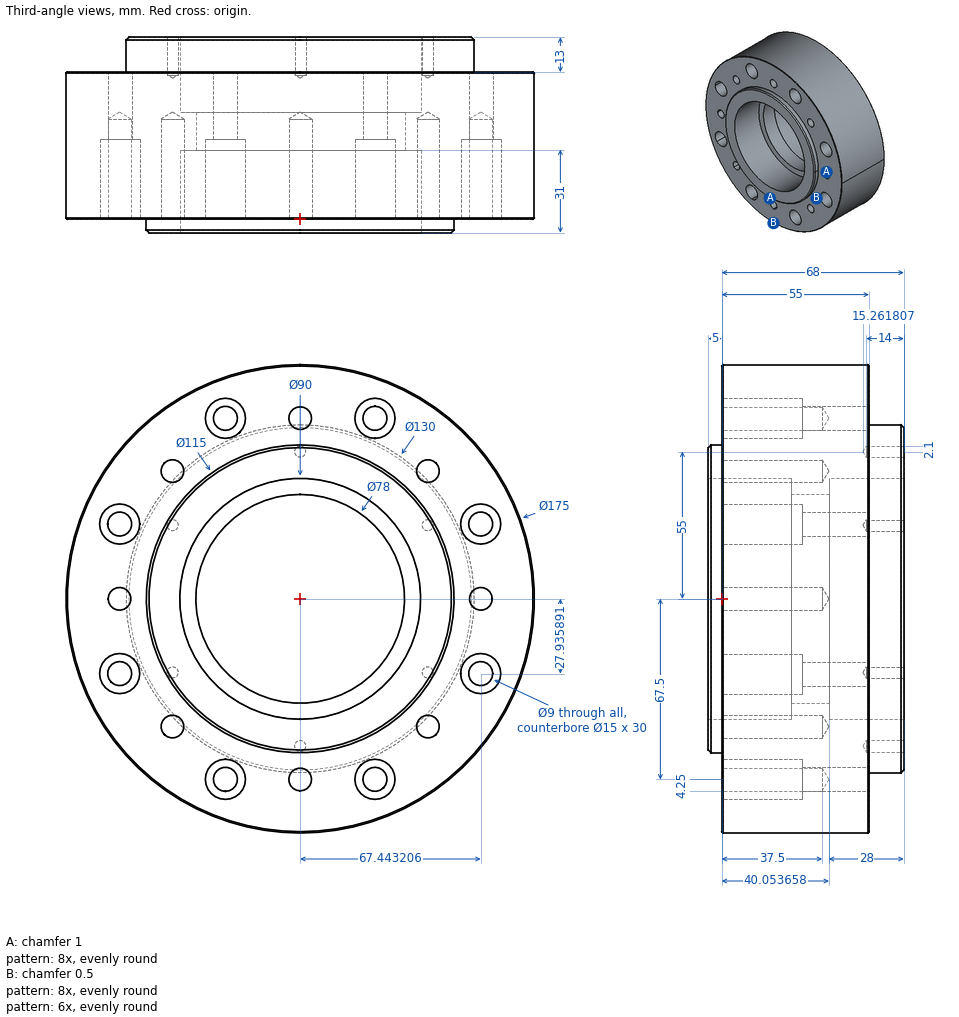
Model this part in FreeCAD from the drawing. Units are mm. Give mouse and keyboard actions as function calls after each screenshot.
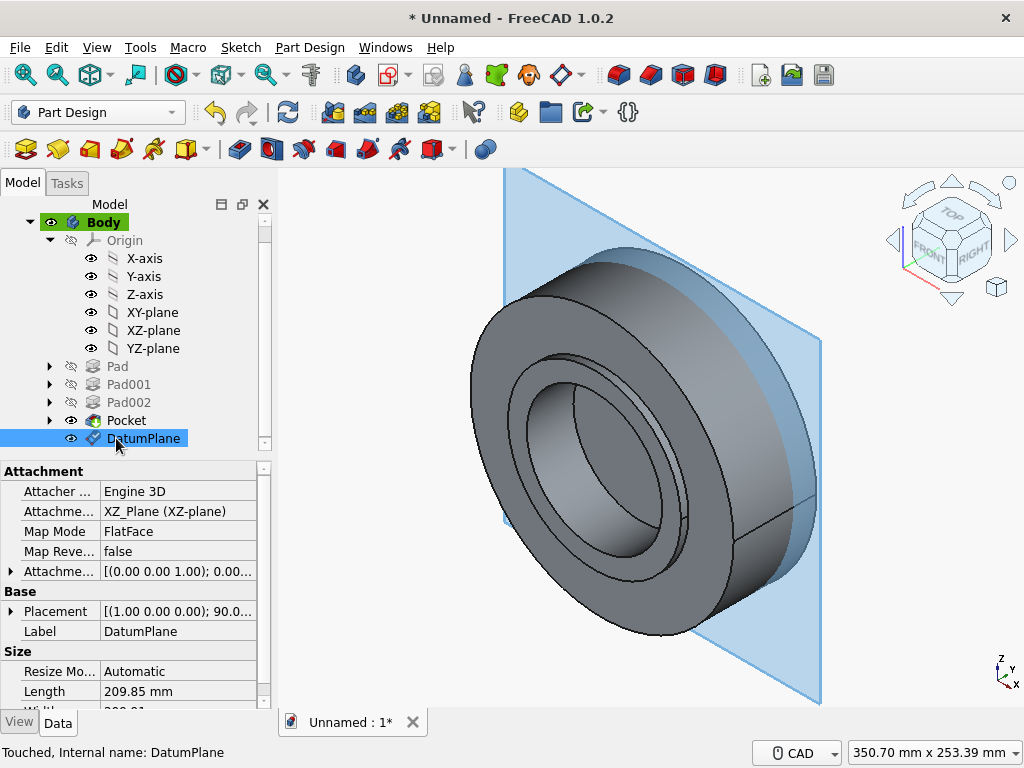
click(388, 76)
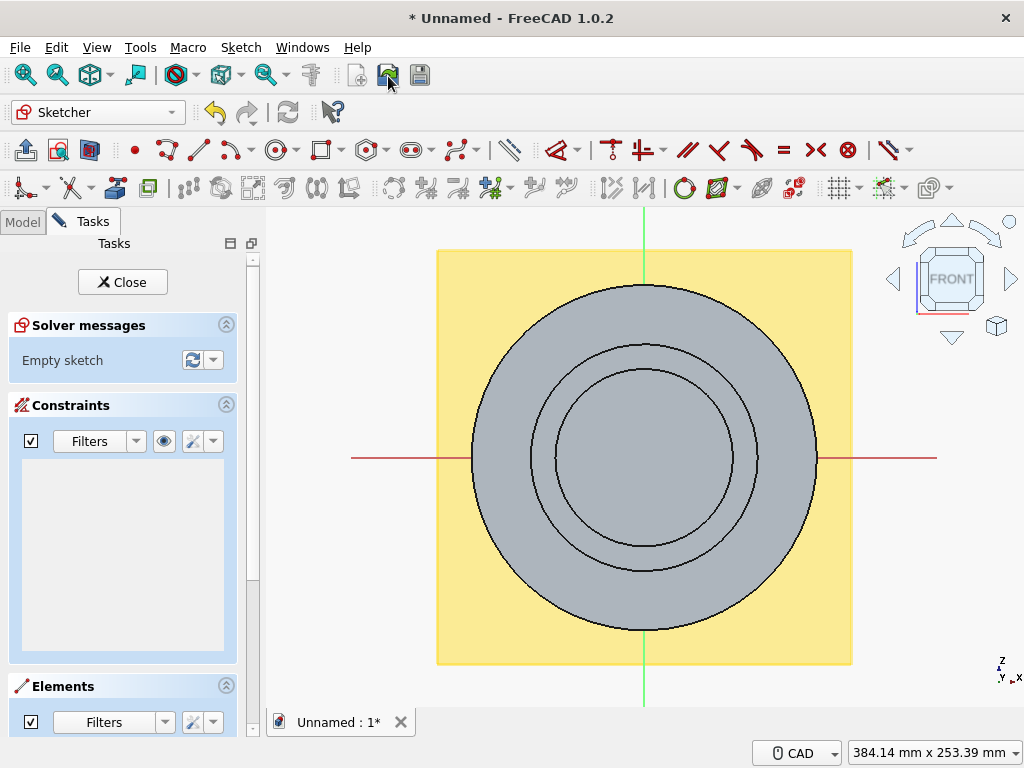
click(90, 150)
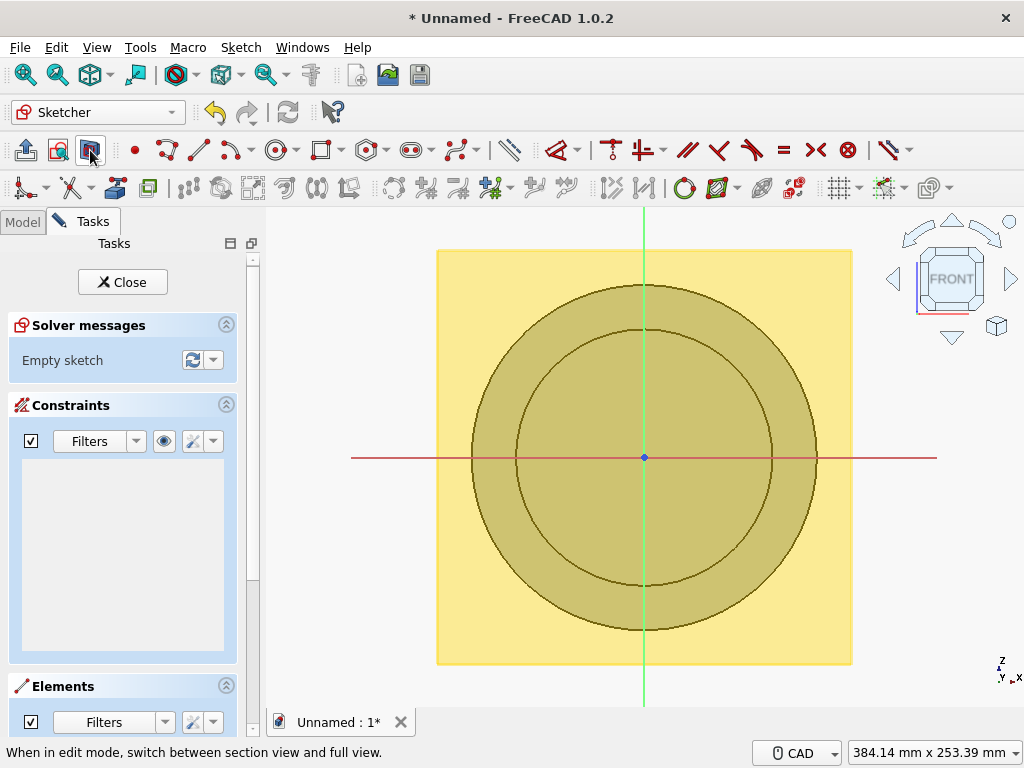
scroll(727, 458, up, 3)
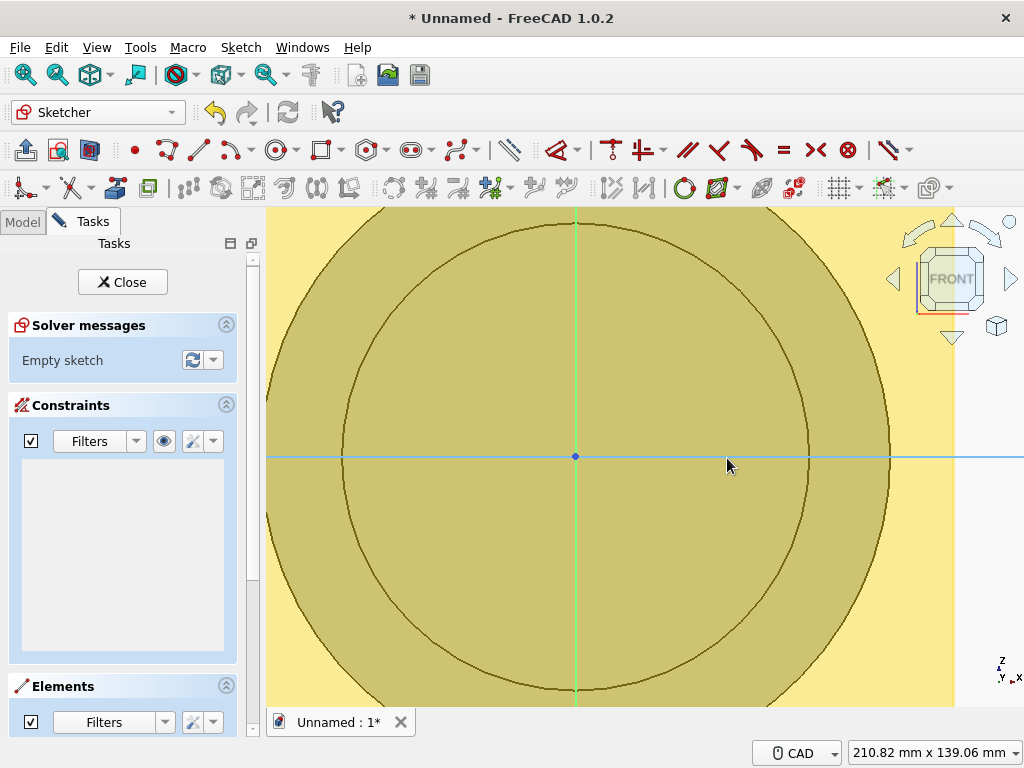
click(276, 150)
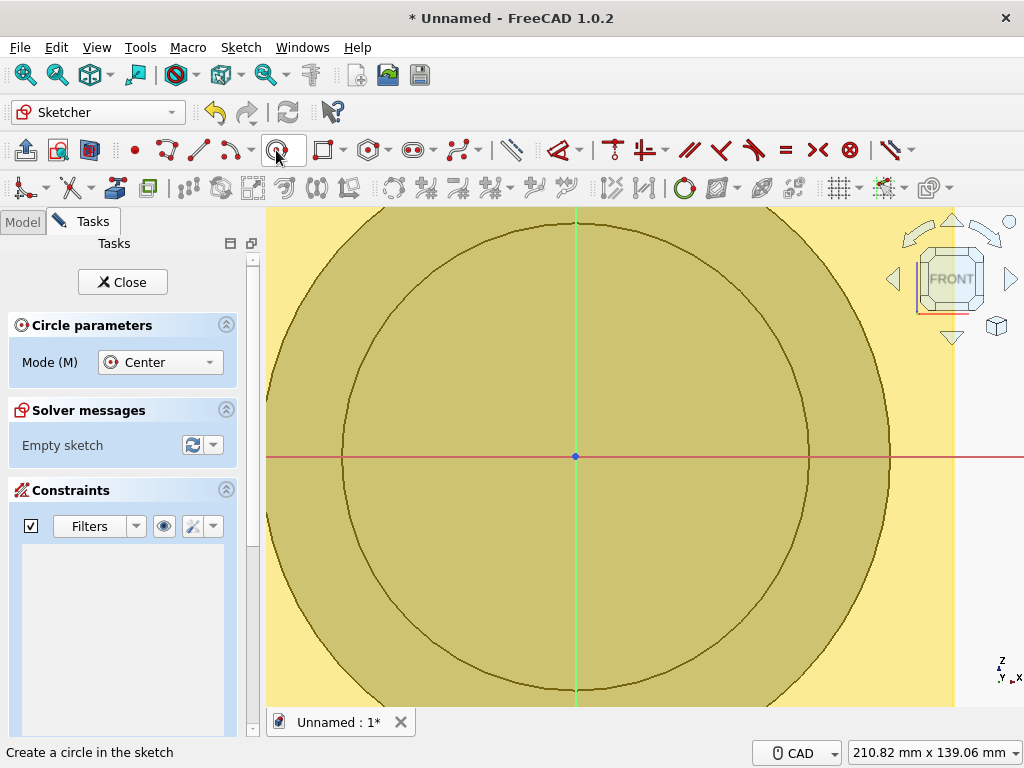
click(576, 457)
click(690, 343)
key(Escape)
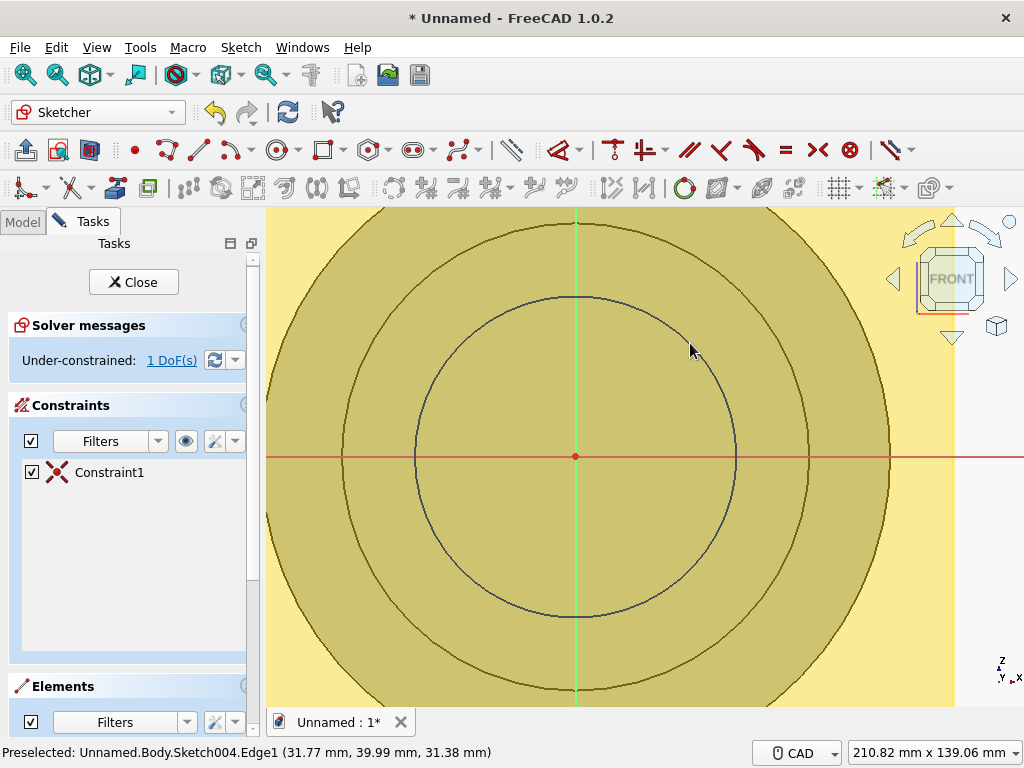
click(558, 150)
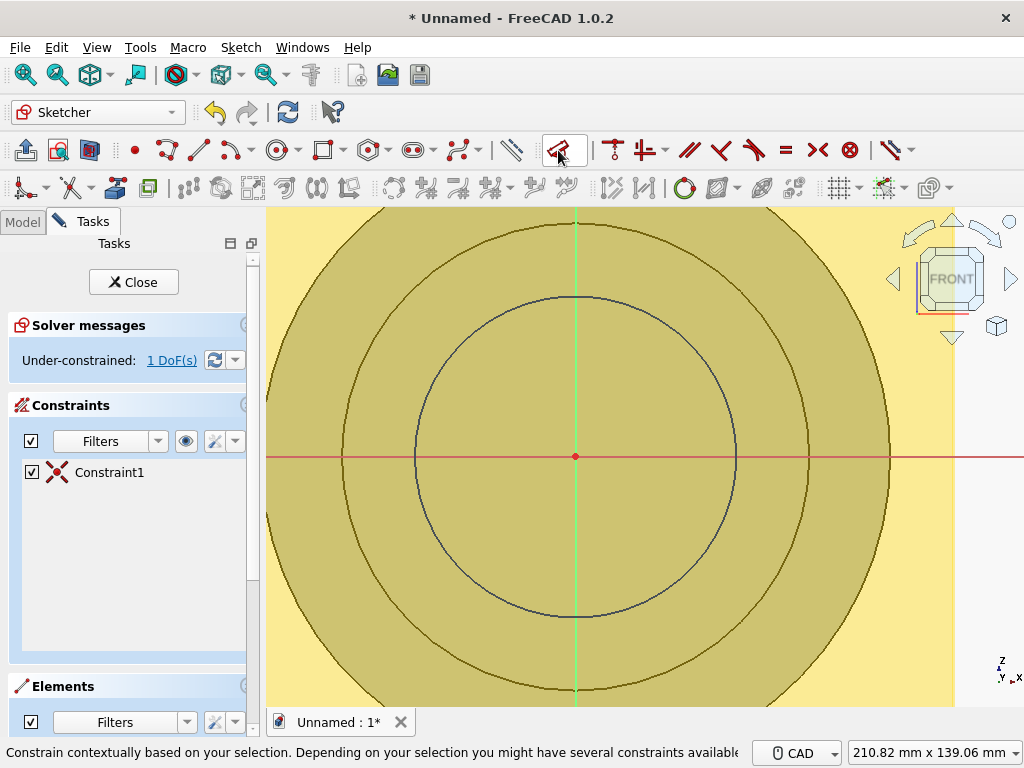
click(689, 343)
click(712, 320)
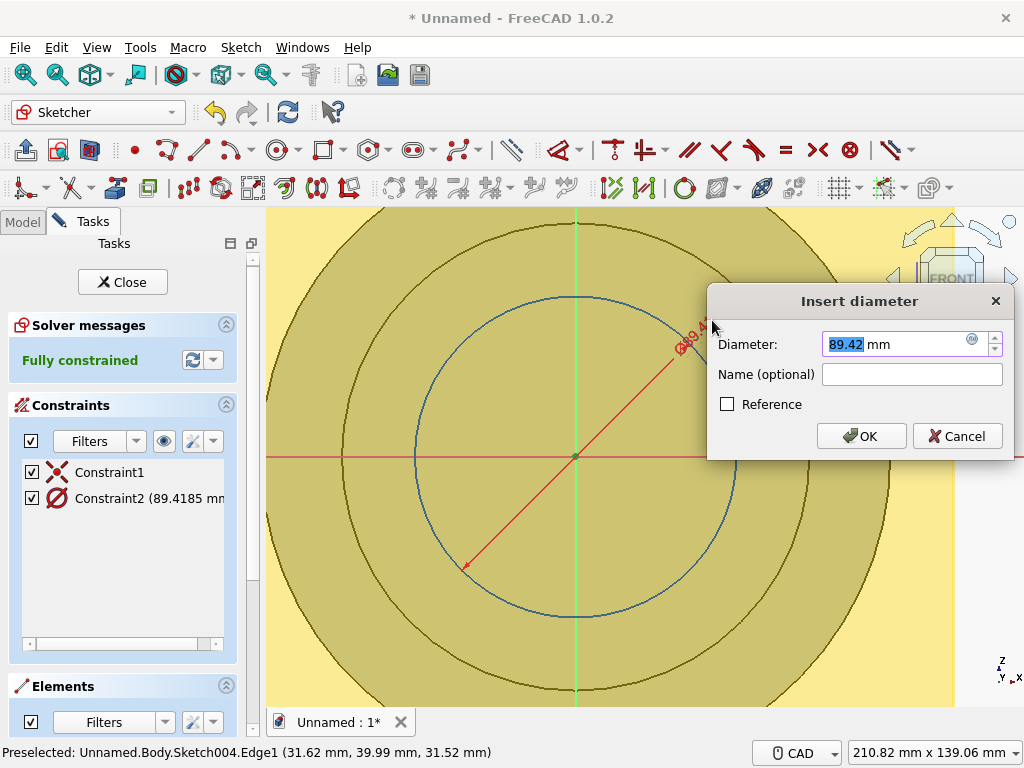
text(90)
key(Return)
key(Escape)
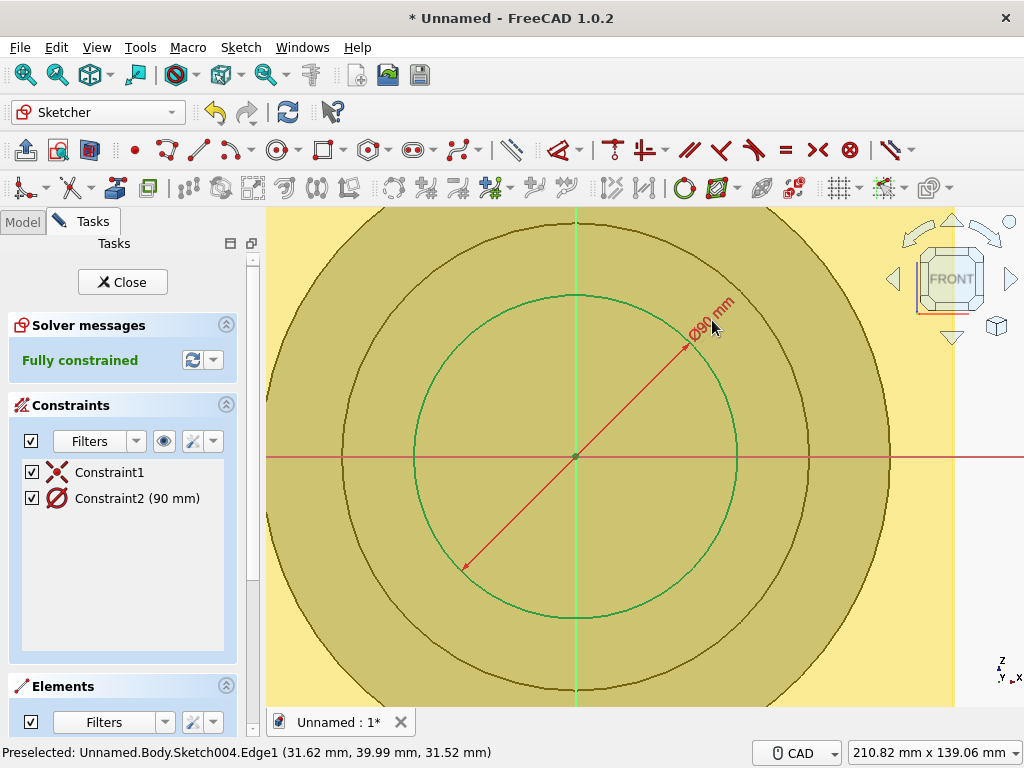
click(123, 282)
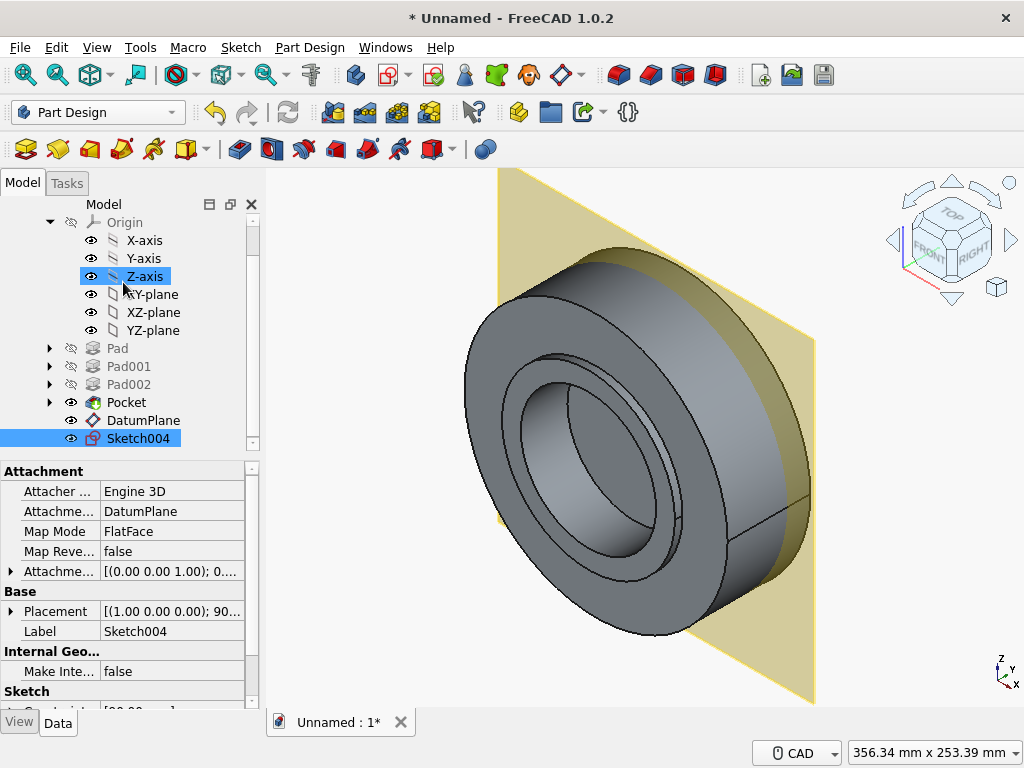
click(240, 150)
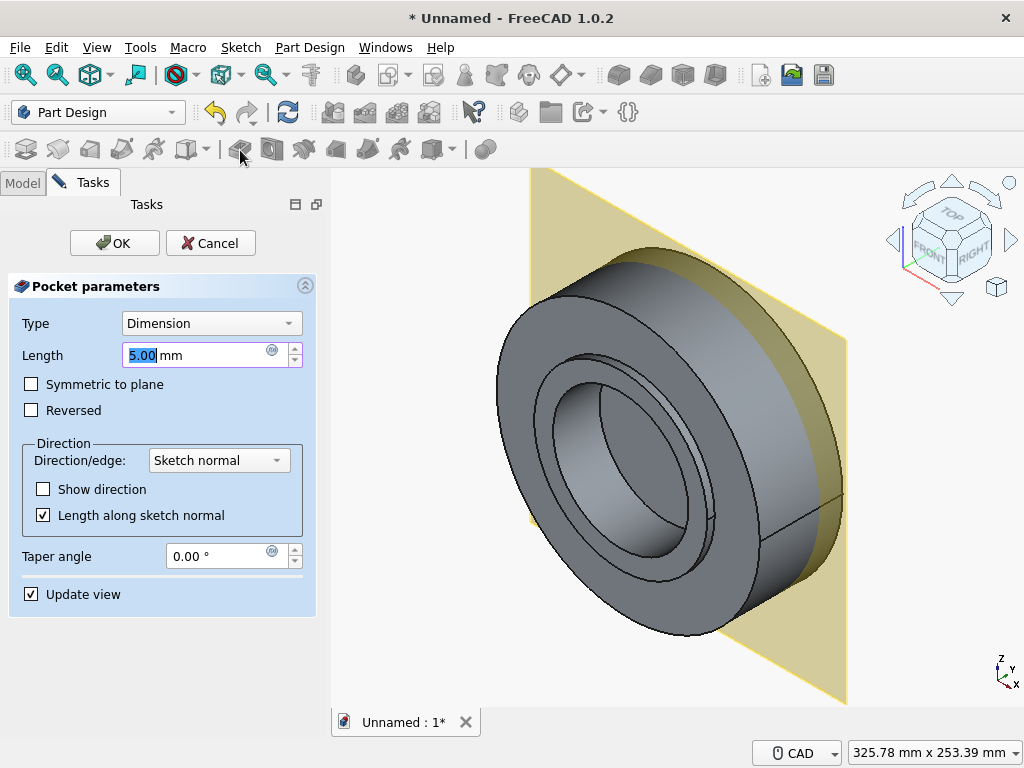
text(28)
key(Tab)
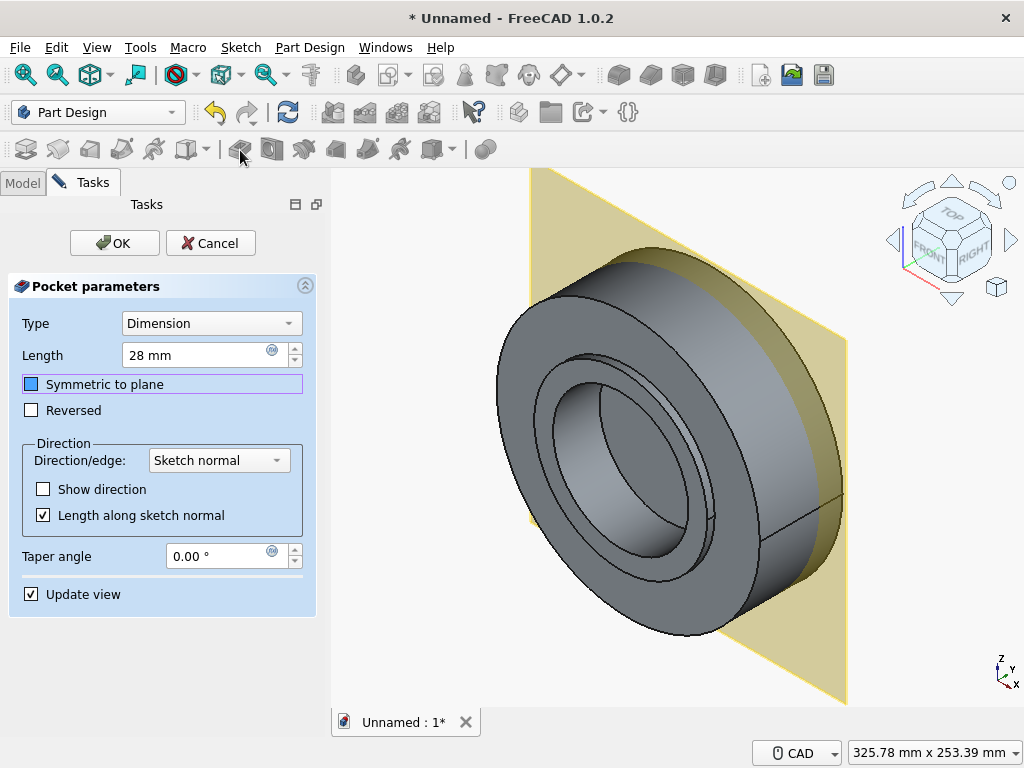
click(115, 243)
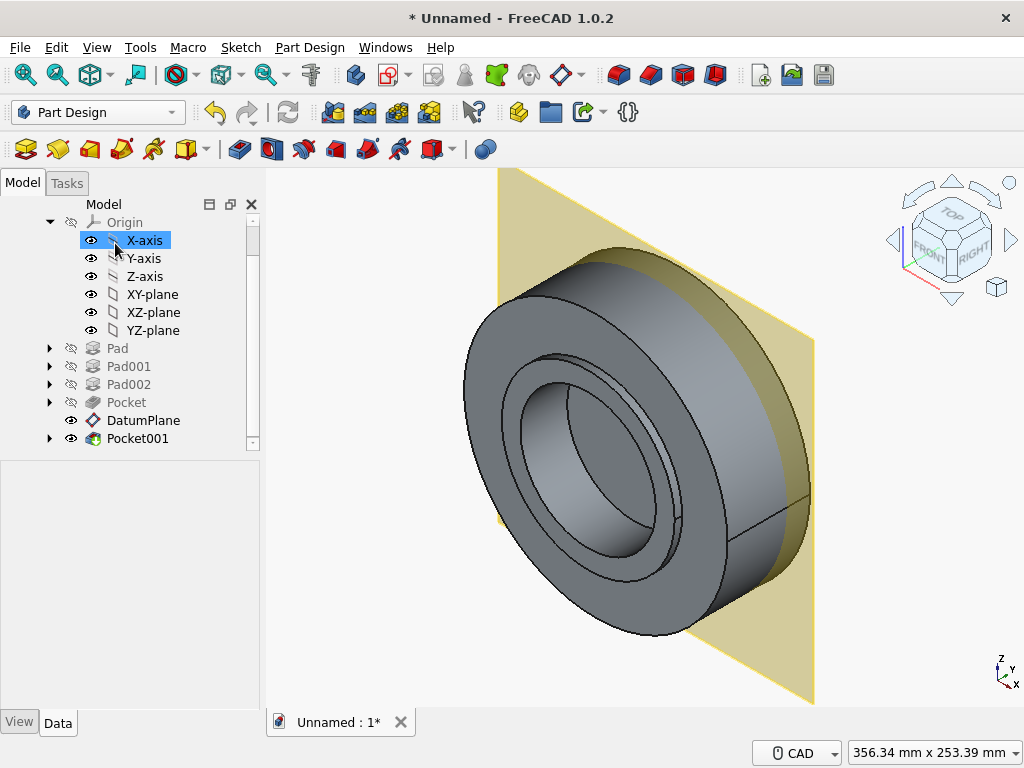
click(116, 420)
key(space)